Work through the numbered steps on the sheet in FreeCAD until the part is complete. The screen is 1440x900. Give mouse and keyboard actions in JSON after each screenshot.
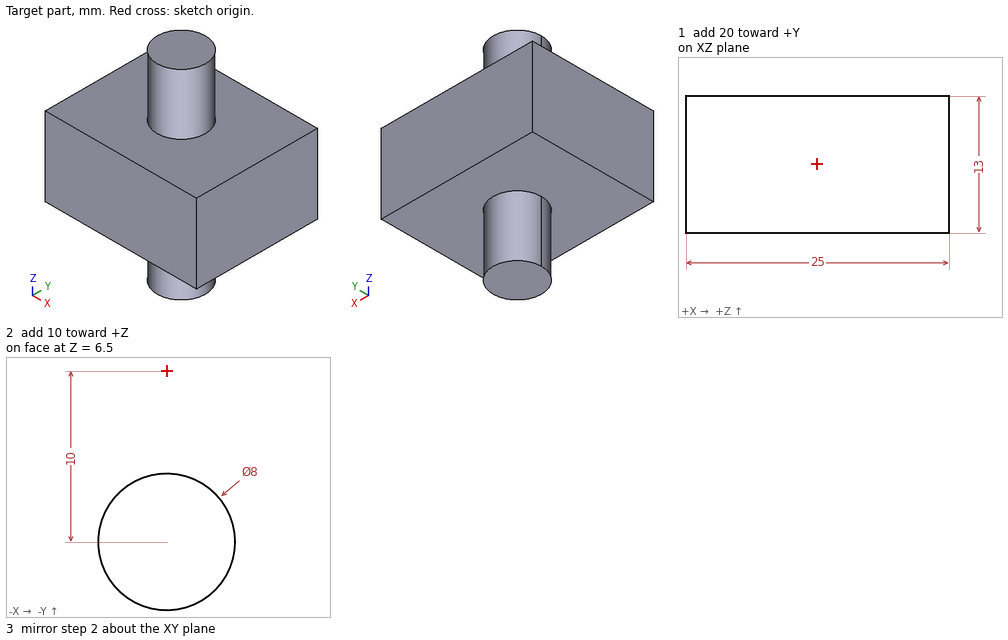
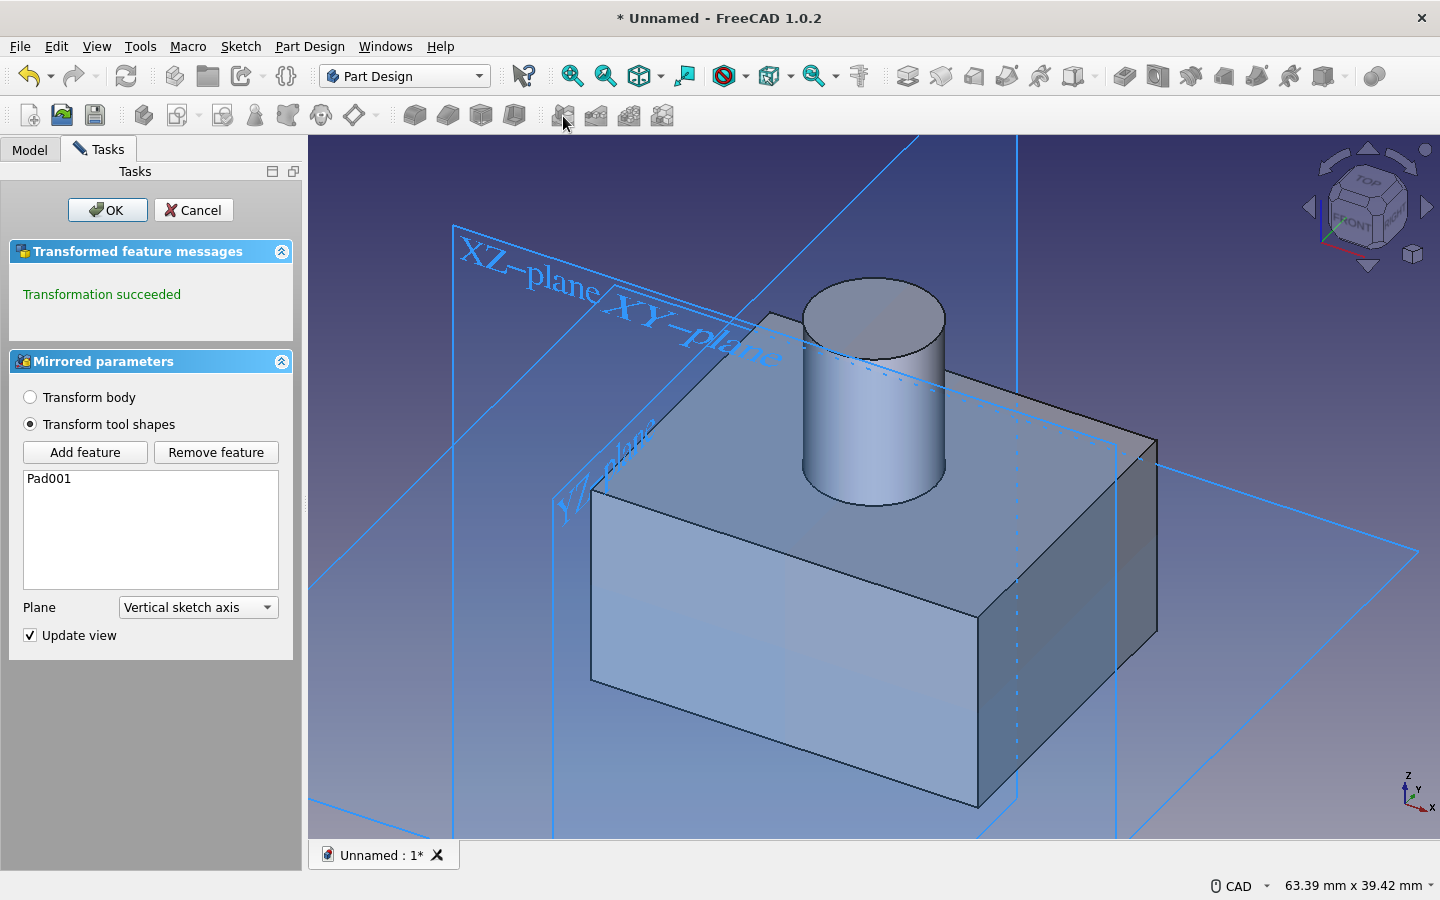
{"action": "left_click", "coordinate": [199, 608]}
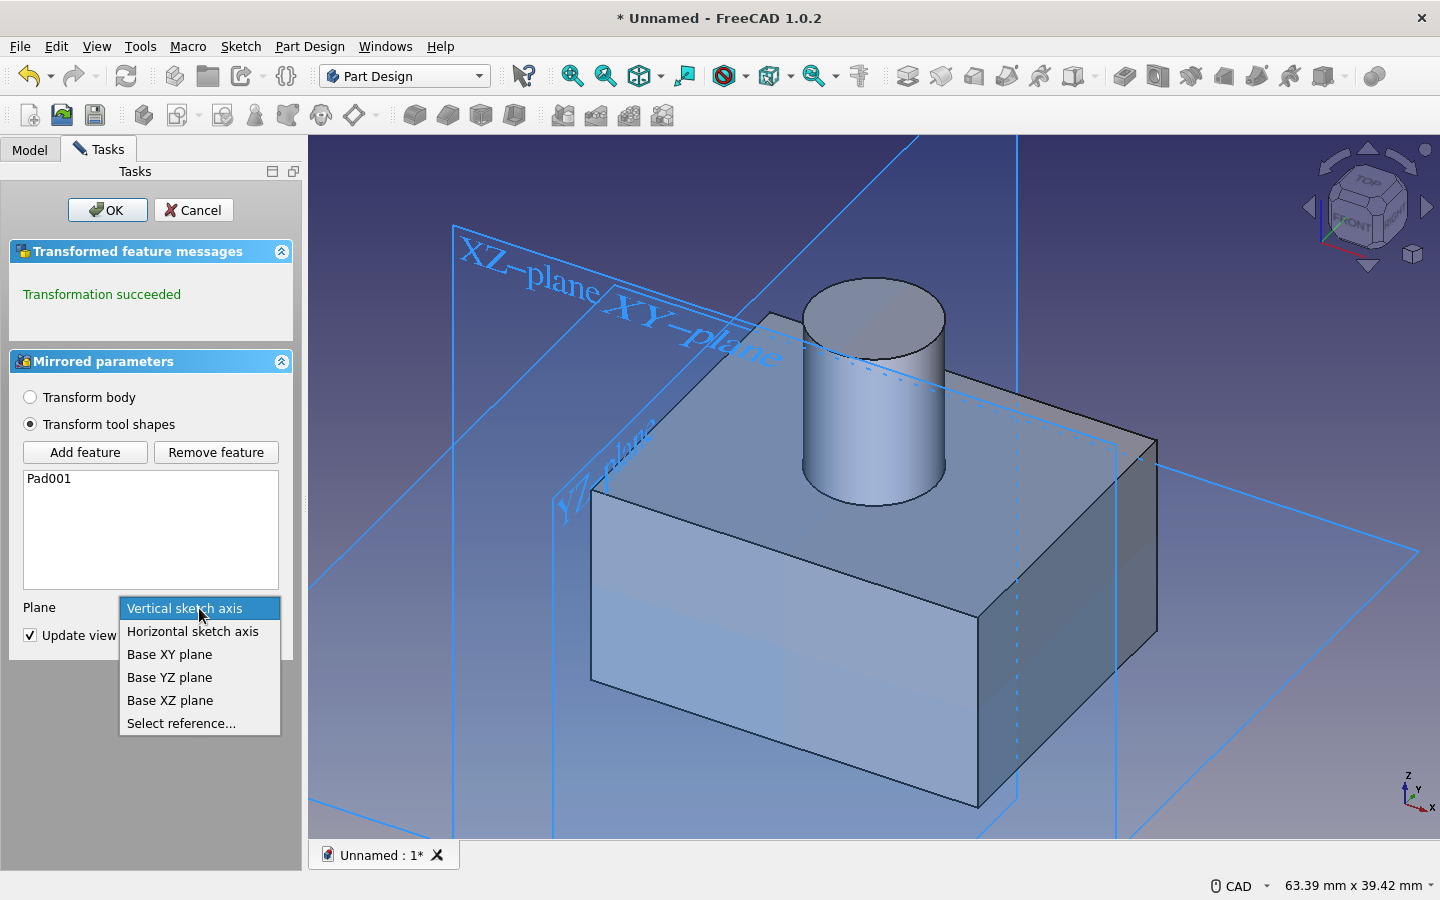
{"action": "left_click", "coordinate": [198, 654]}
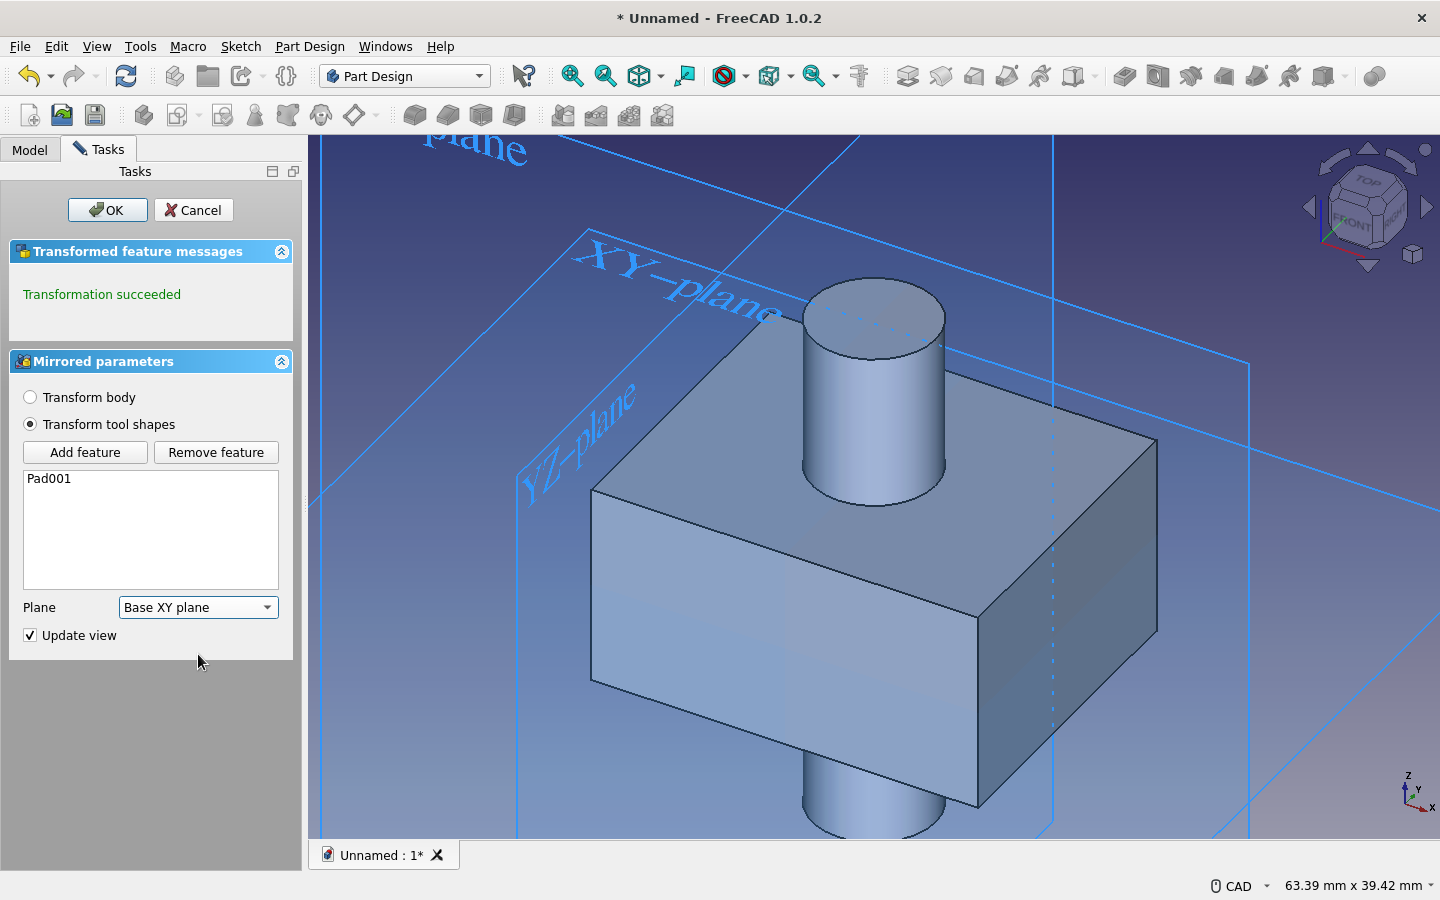
{"action": "left_click", "coordinate": [108, 210]}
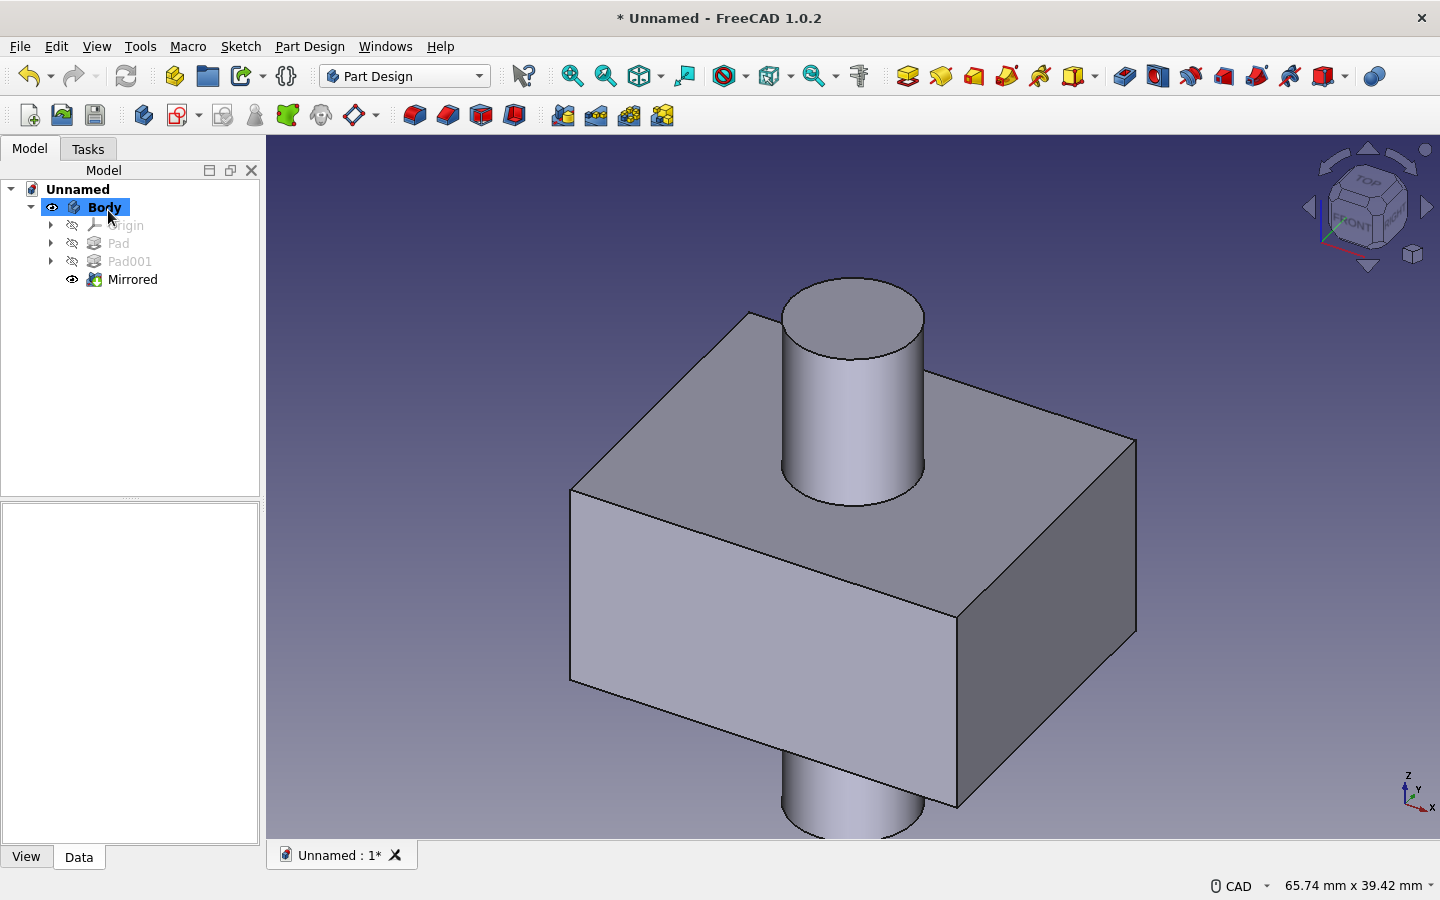
{"action": "key", "text": "0"}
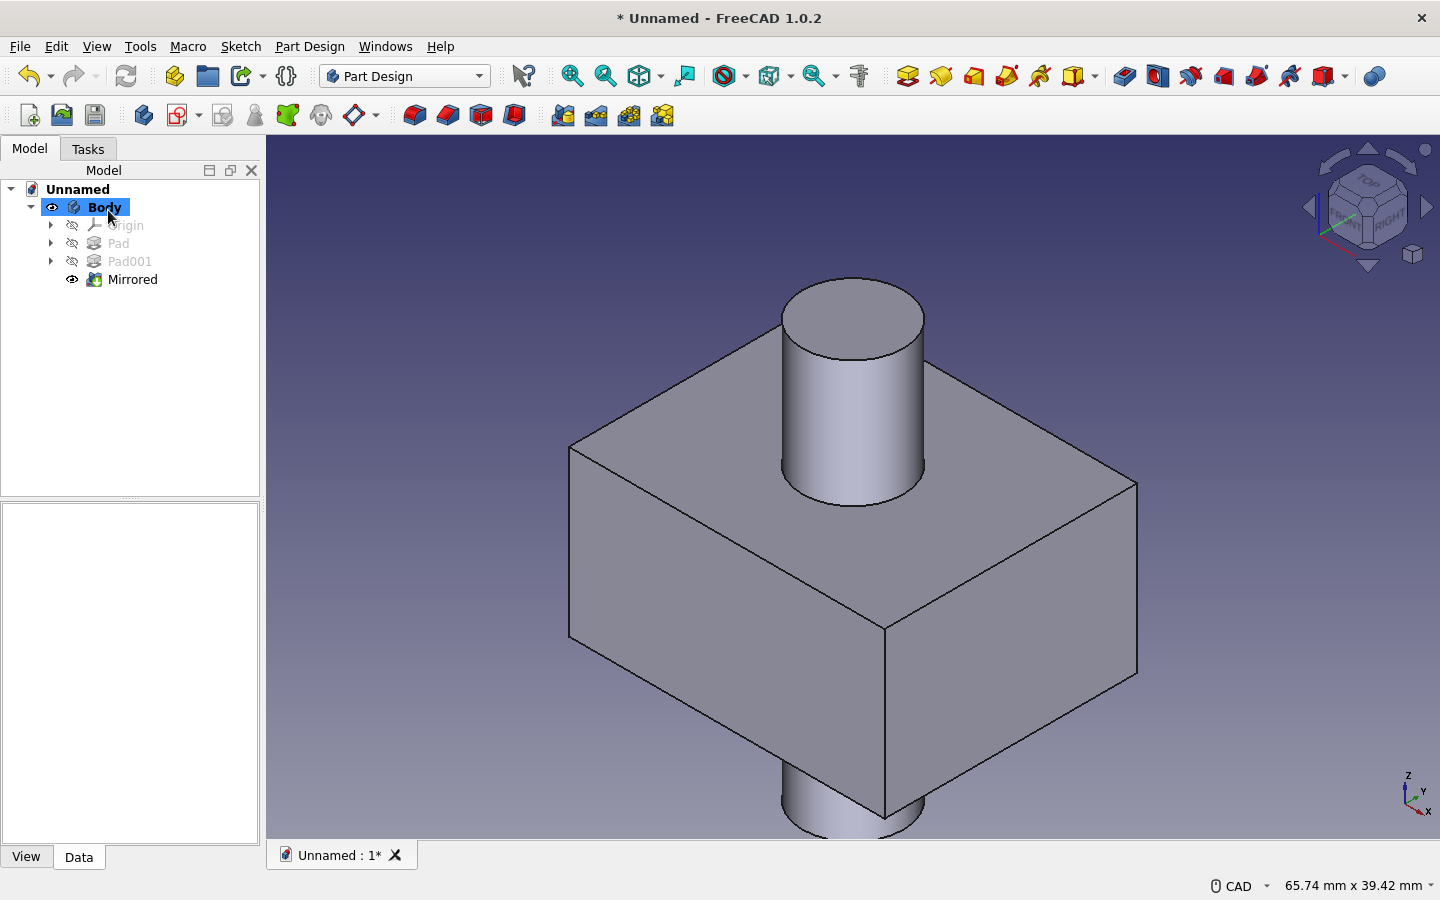
{"action": "key", "text": "v f"}